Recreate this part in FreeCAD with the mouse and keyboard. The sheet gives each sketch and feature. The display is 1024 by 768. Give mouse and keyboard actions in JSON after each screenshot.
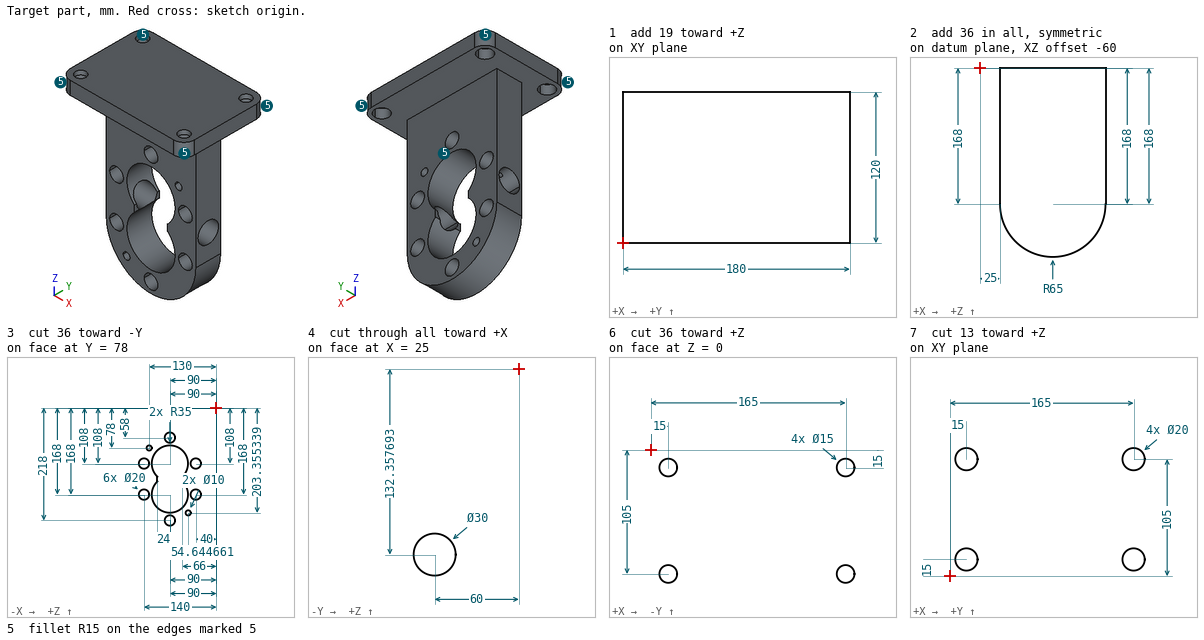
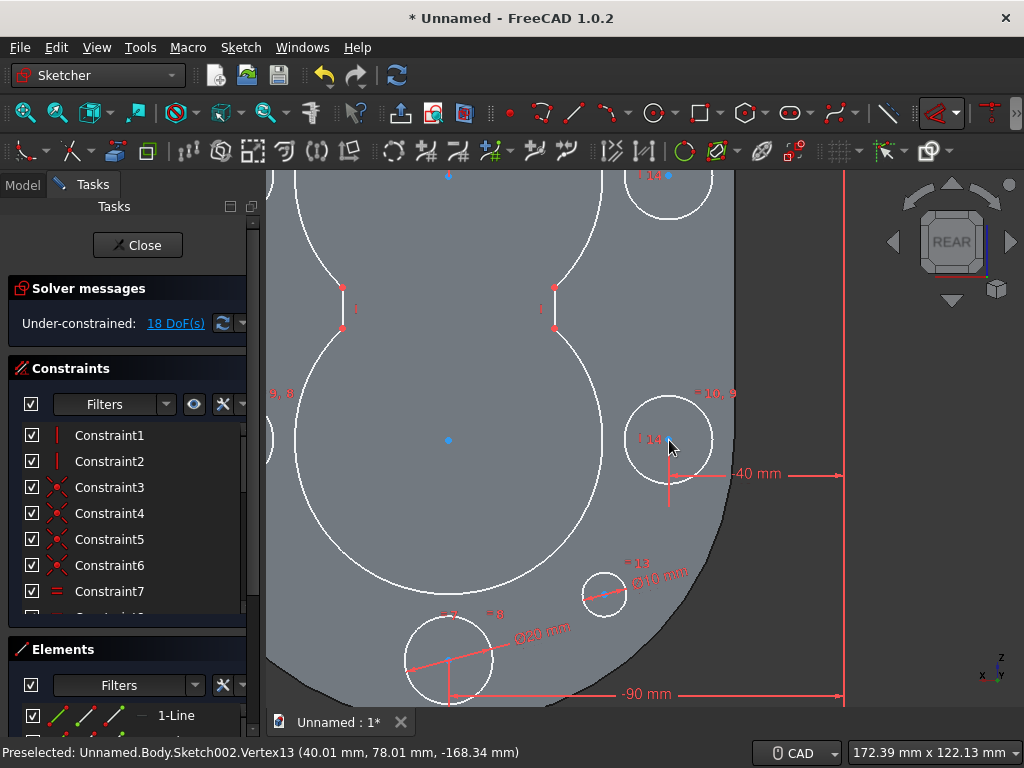
{"action": "scroll", "coordinate": [612, 577], "scroll_direction": "down", "scroll_amount": 5}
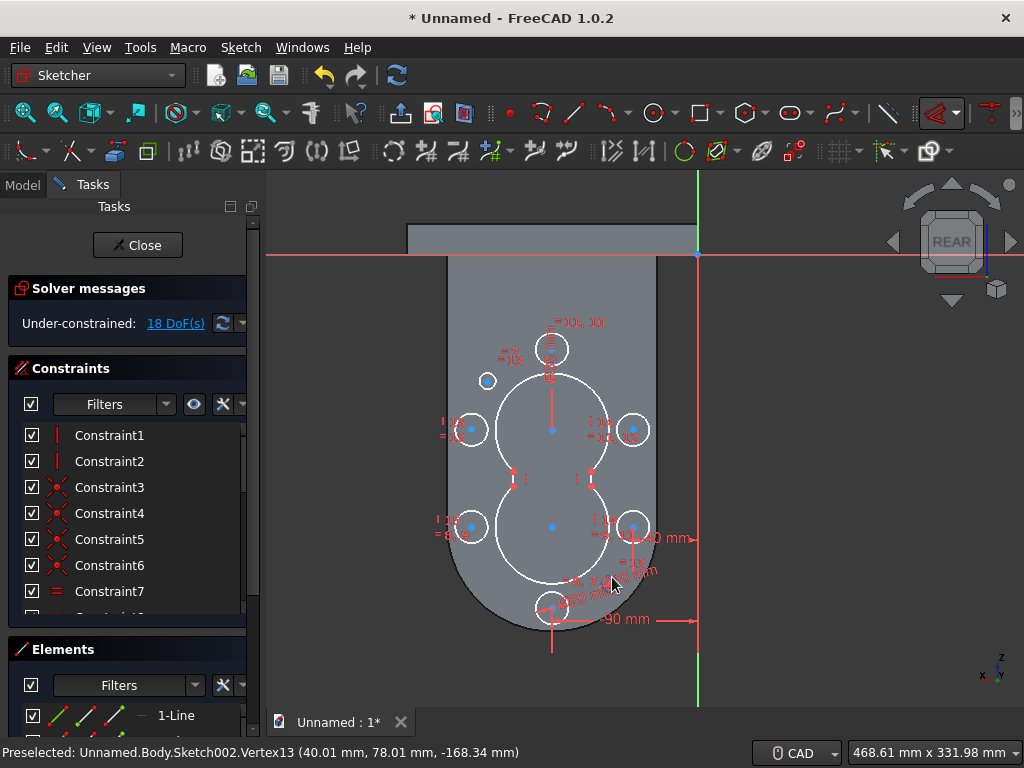
{"action": "left_click", "coordinate": [552, 349]}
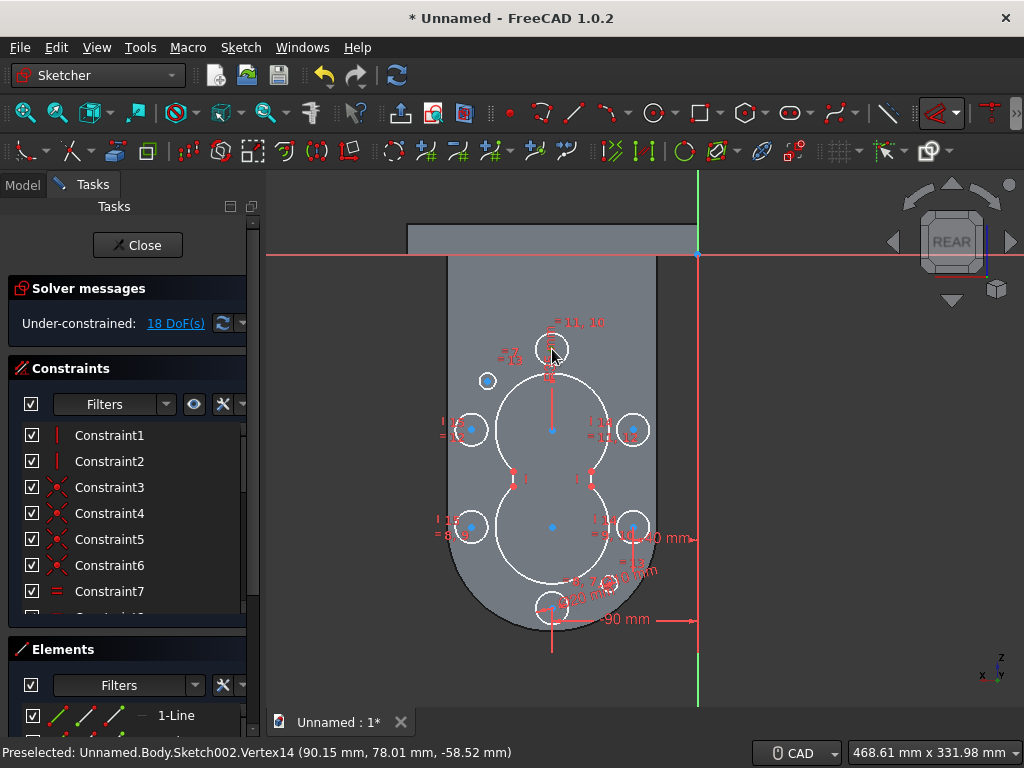
{"action": "left_click", "coordinate": [958, 114]}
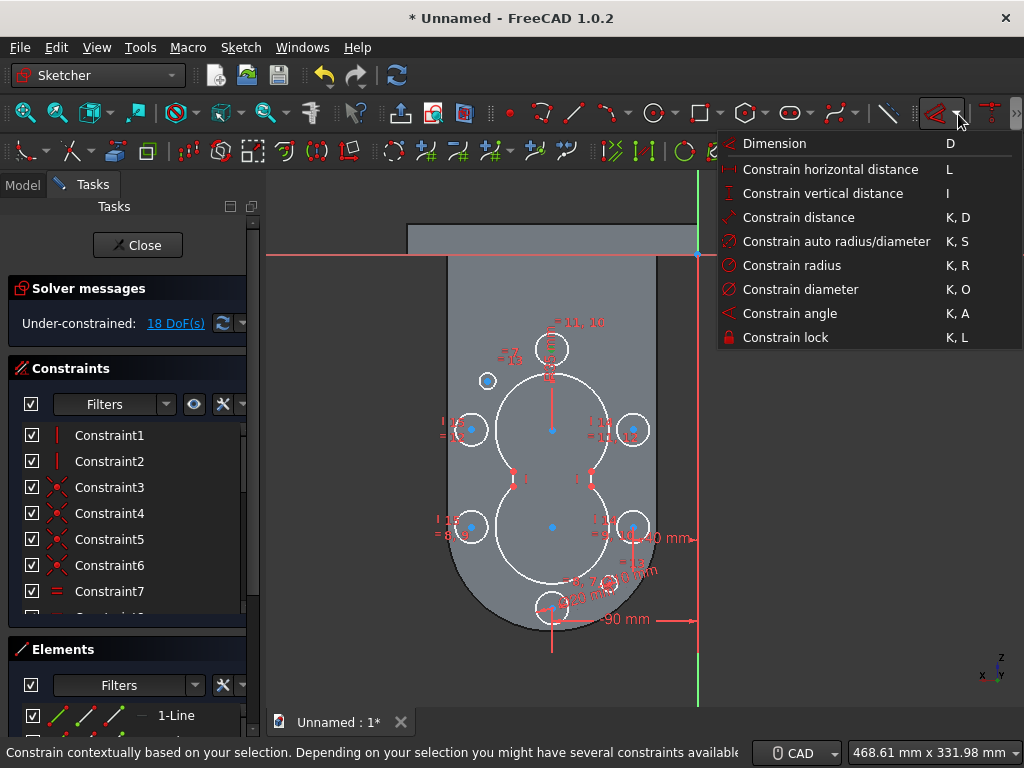
{"action": "left_click", "coordinate": [870, 169]}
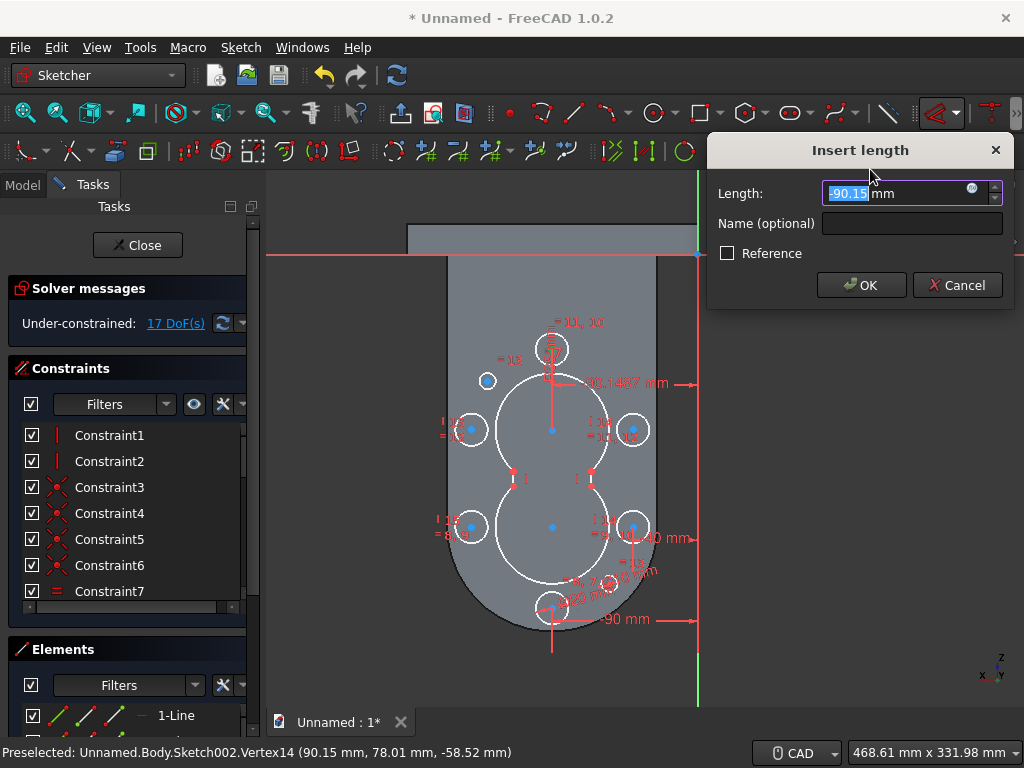
{"action": "type", "text": "-90"}
{"action": "key", "text": "Return"}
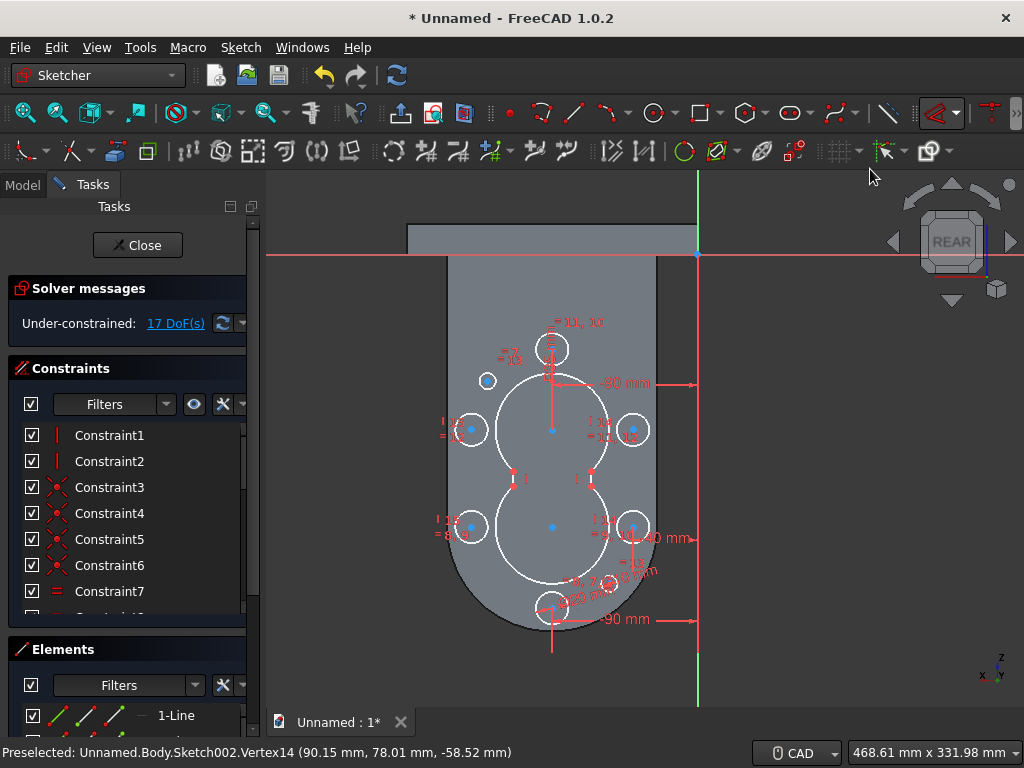
{"action": "left_click", "coordinate": [552, 349]}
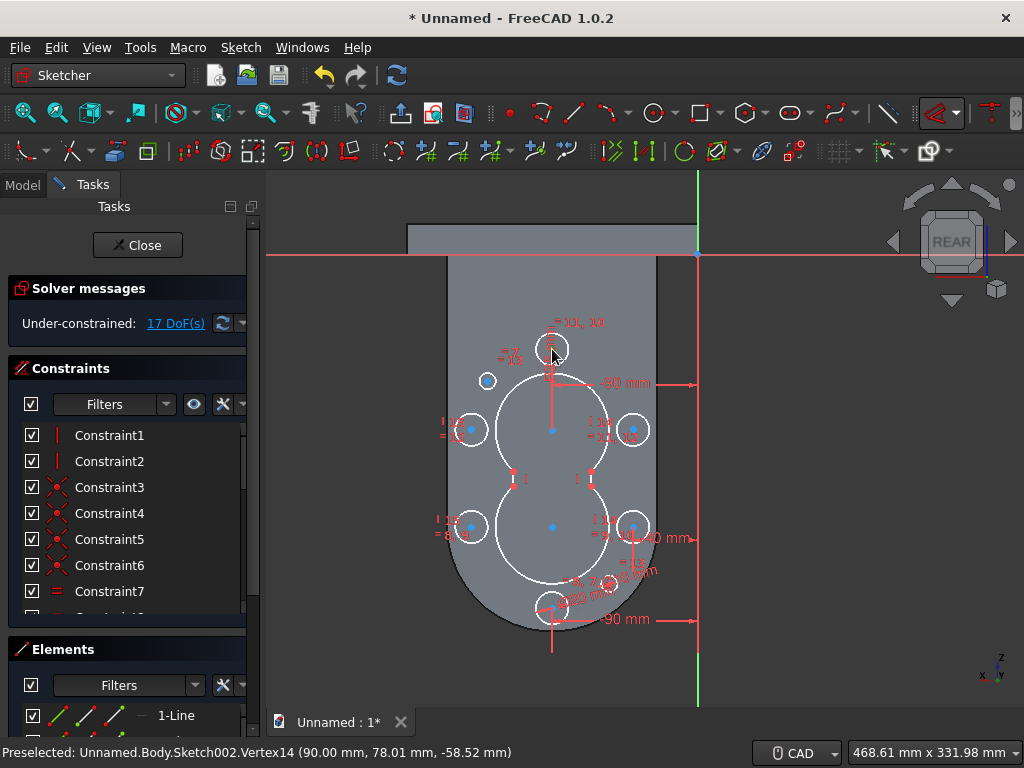
{"action": "left_click", "coordinate": [958, 114]}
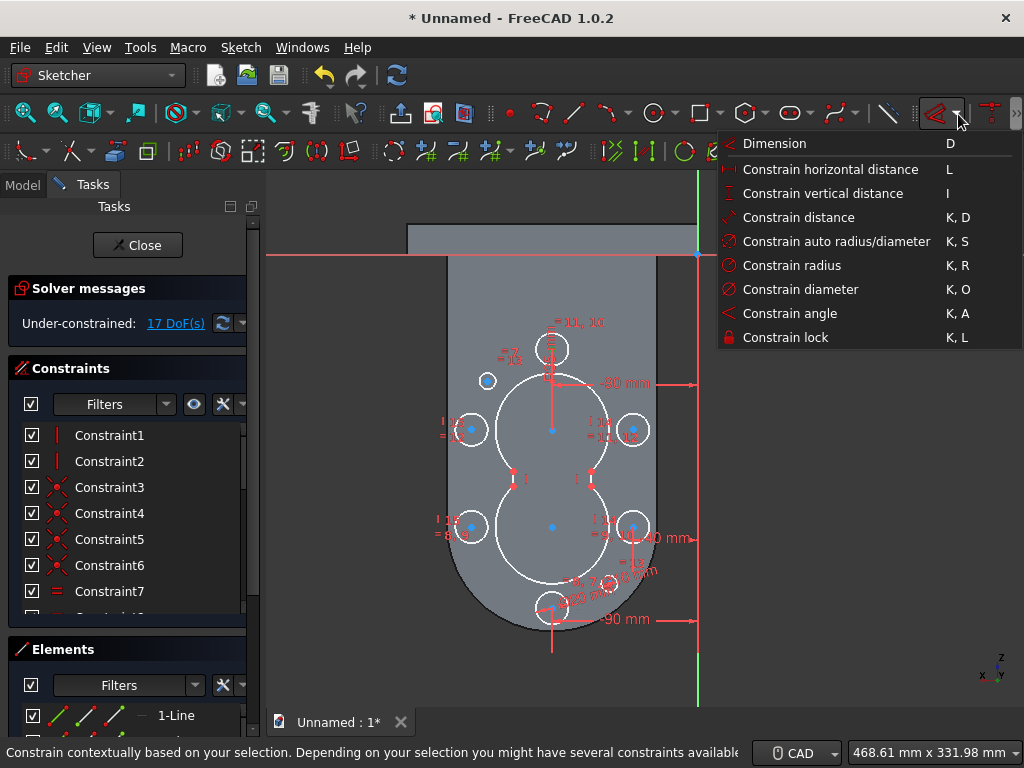
{"action": "left_click", "coordinate": [870, 193]}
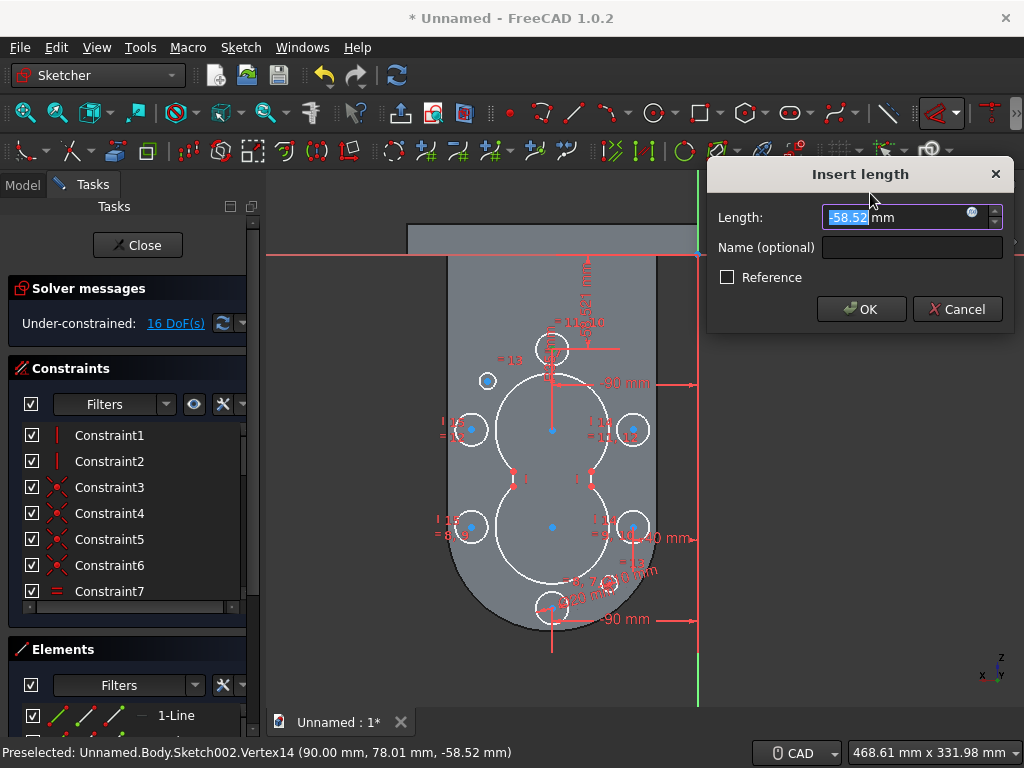
{"action": "type", "text": "-58"}
{"action": "key", "text": "Return"}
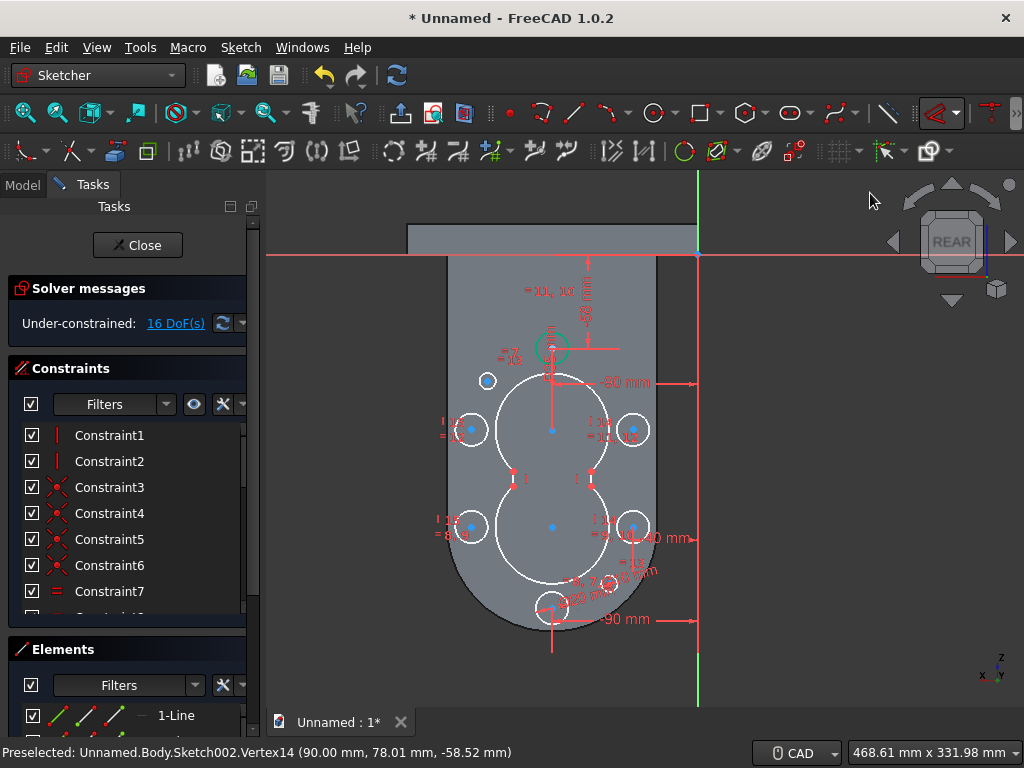
{"action": "left_click", "coordinate": [488, 381]}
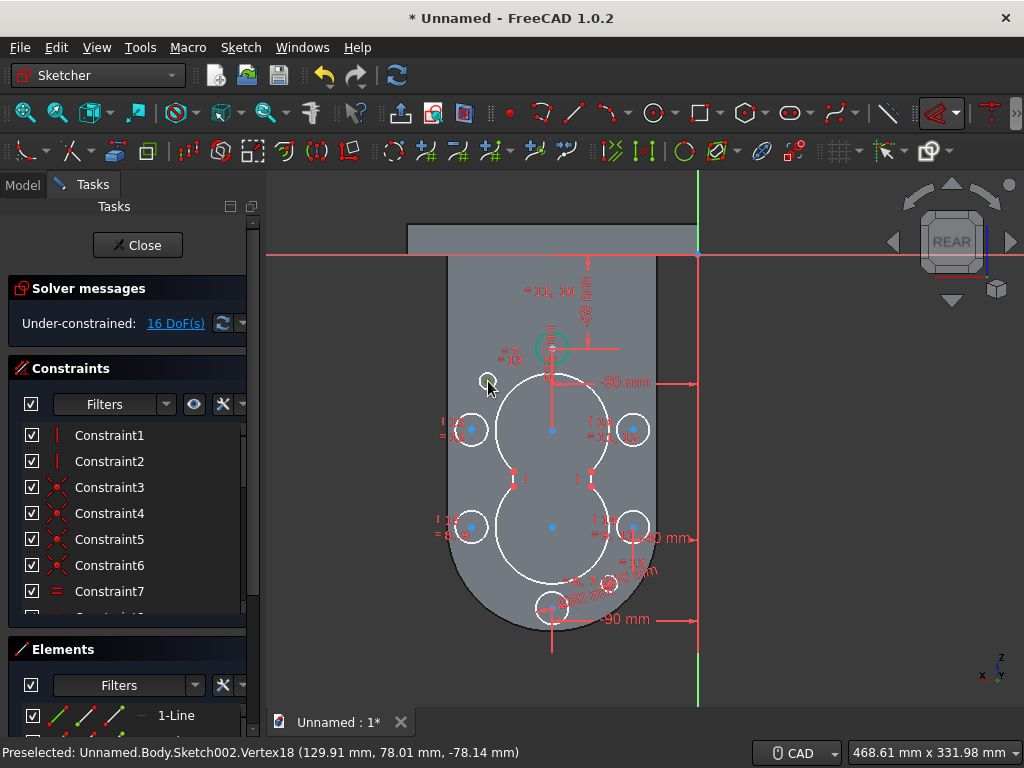
{"action": "key", "text": "i"}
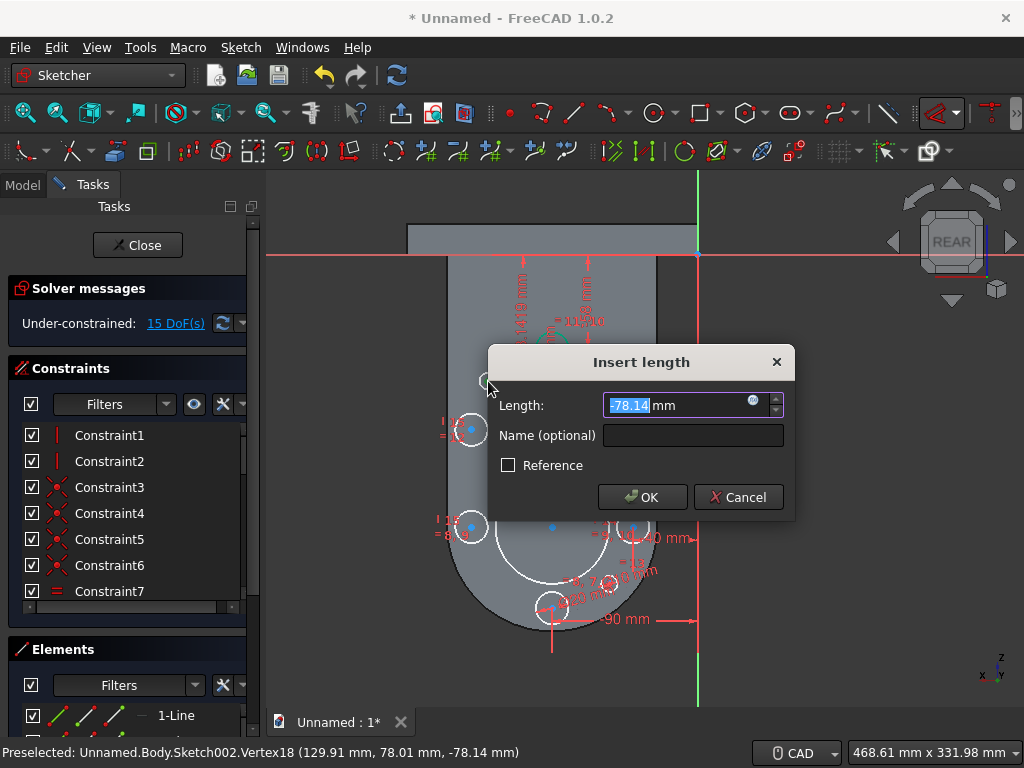
{"action": "type", "text": "-78"}
{"action": "key", "text": "Return"}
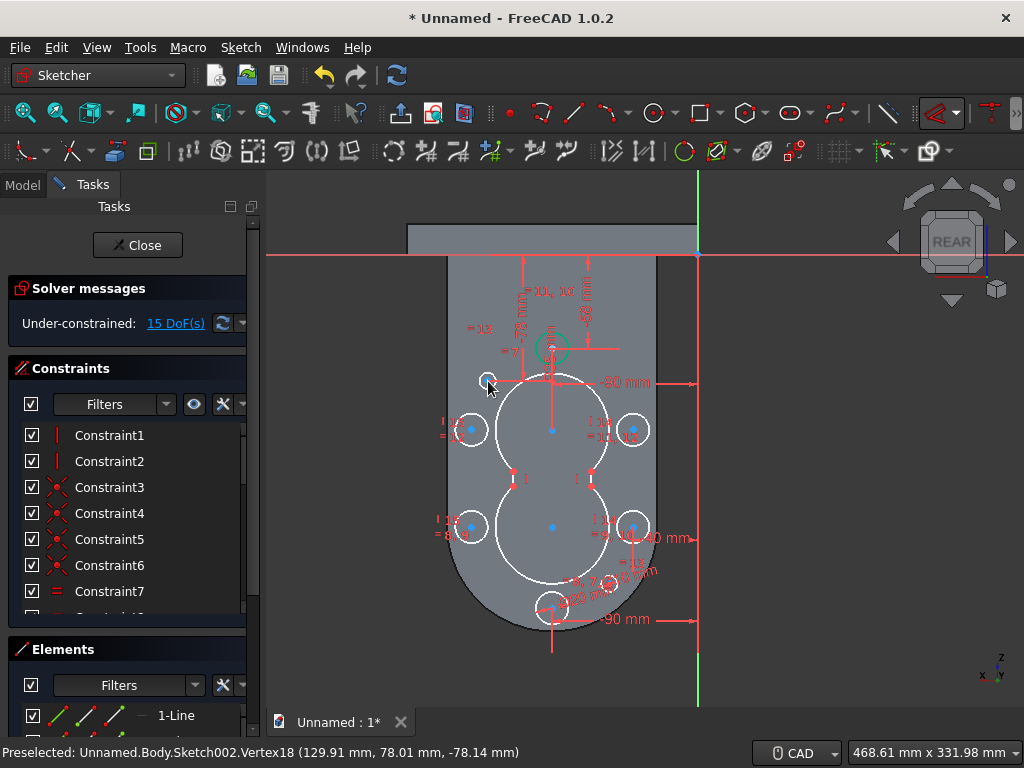
{"action": "left_click", "coordinate": [591, 486]}